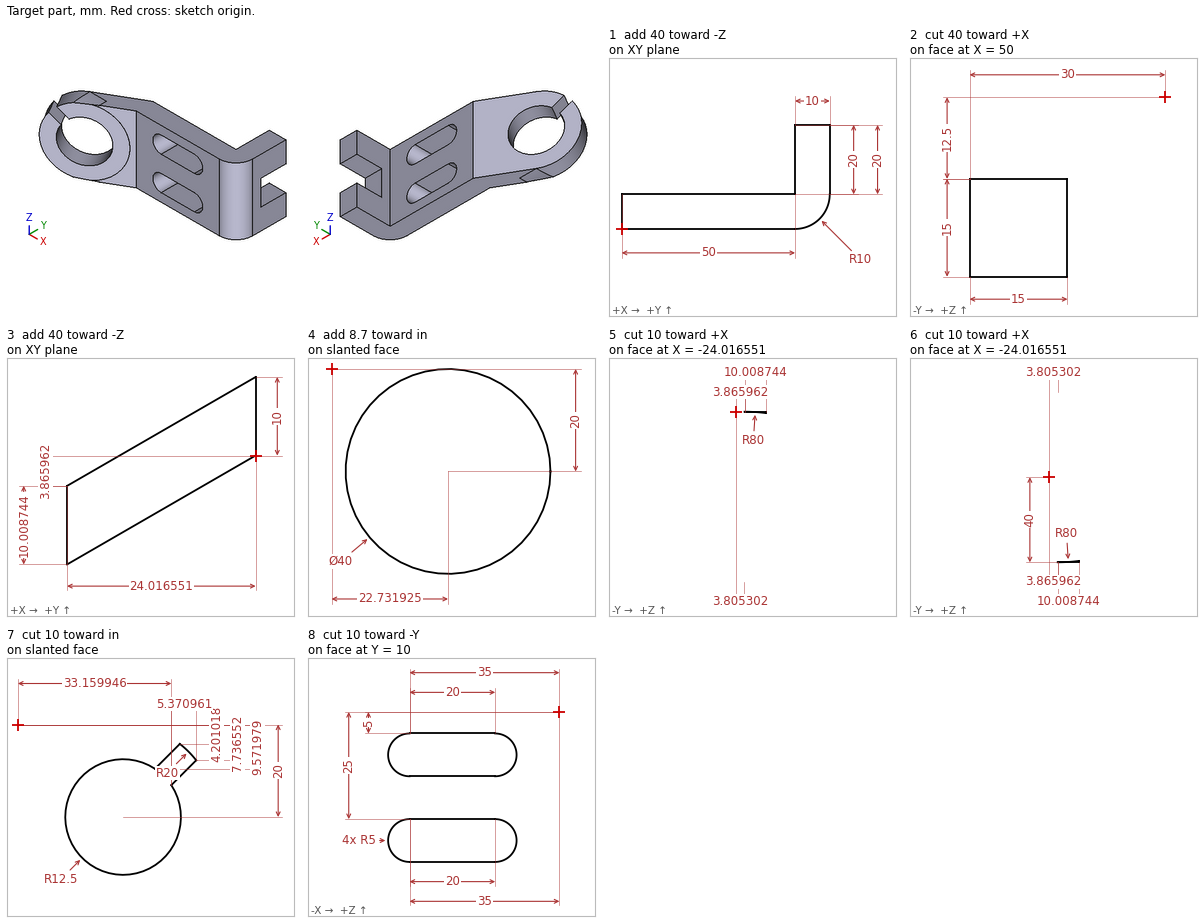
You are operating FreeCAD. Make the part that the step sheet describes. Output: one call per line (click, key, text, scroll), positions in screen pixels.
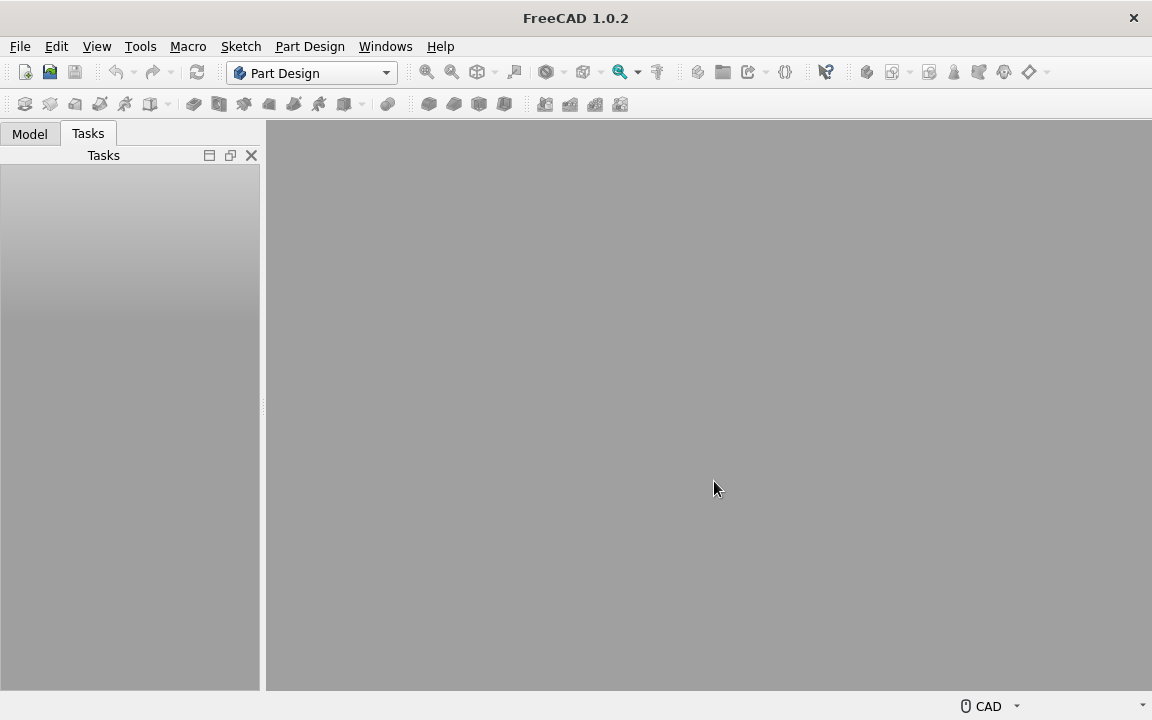
click(25, 72)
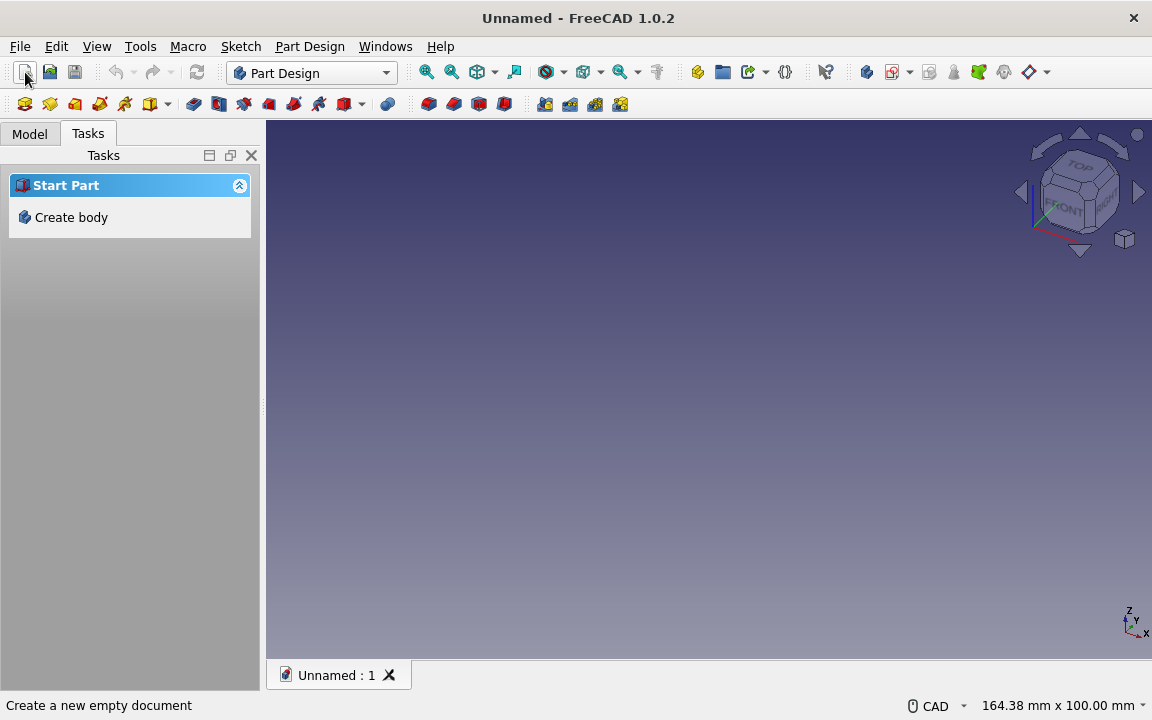
click(892, 72)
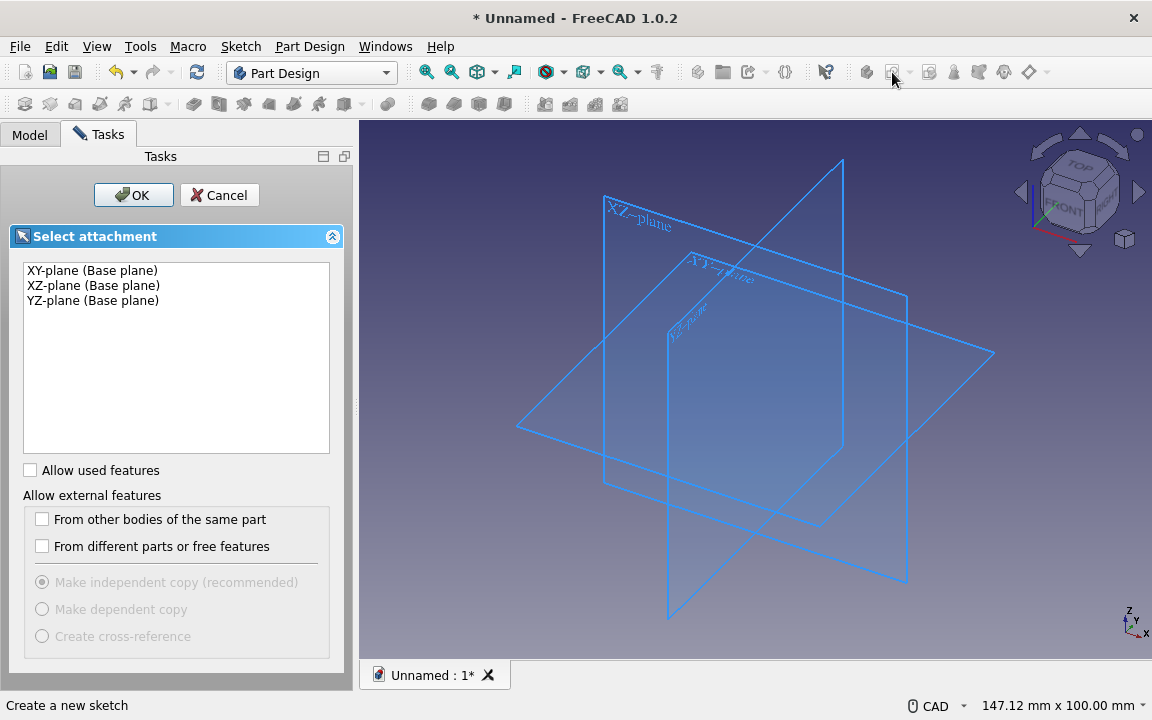
click(84, 270)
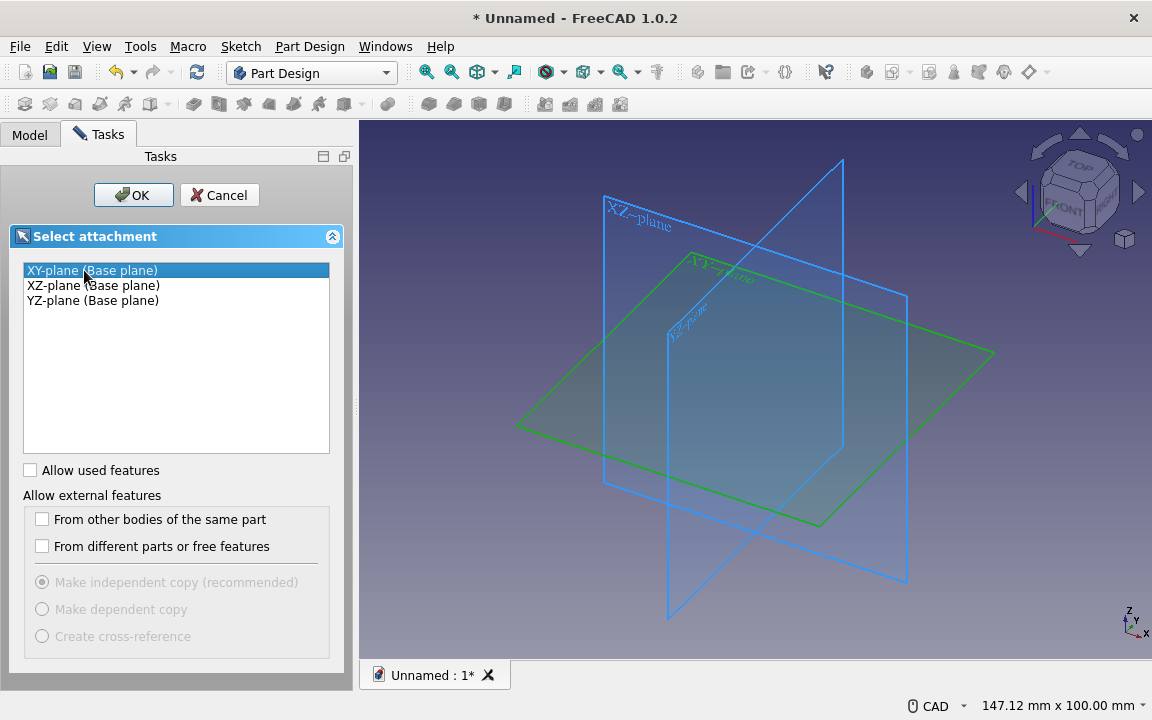
click(134, 195)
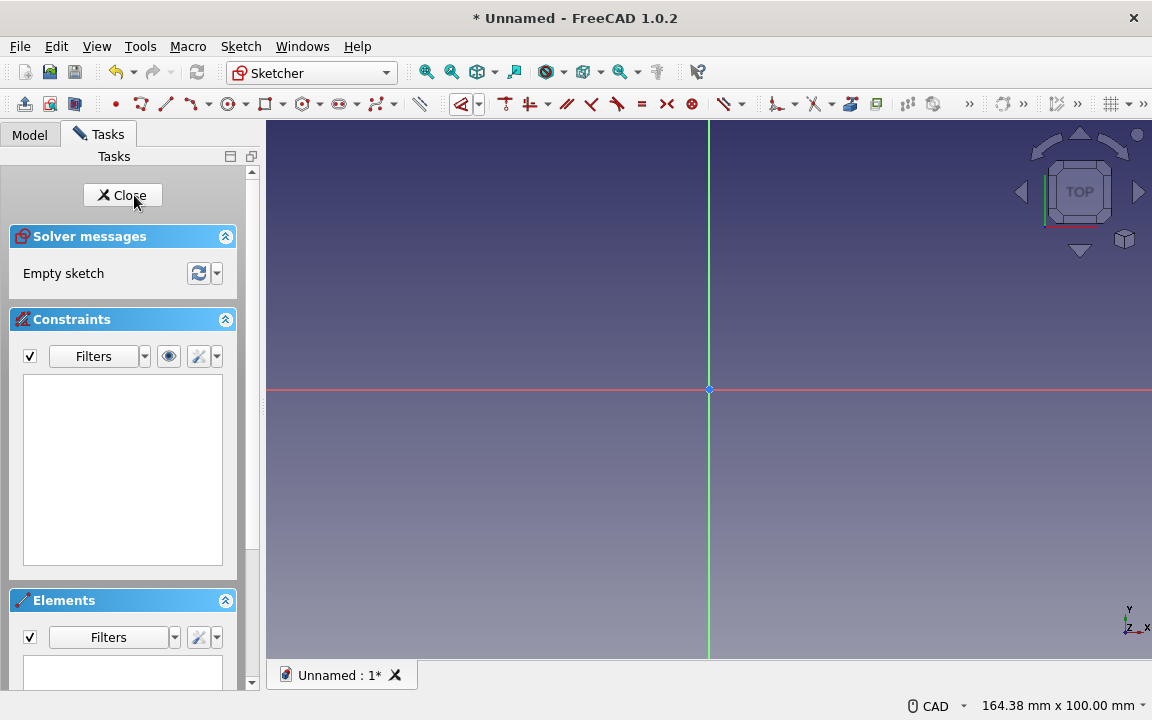
scroll(294, 631, down, 1)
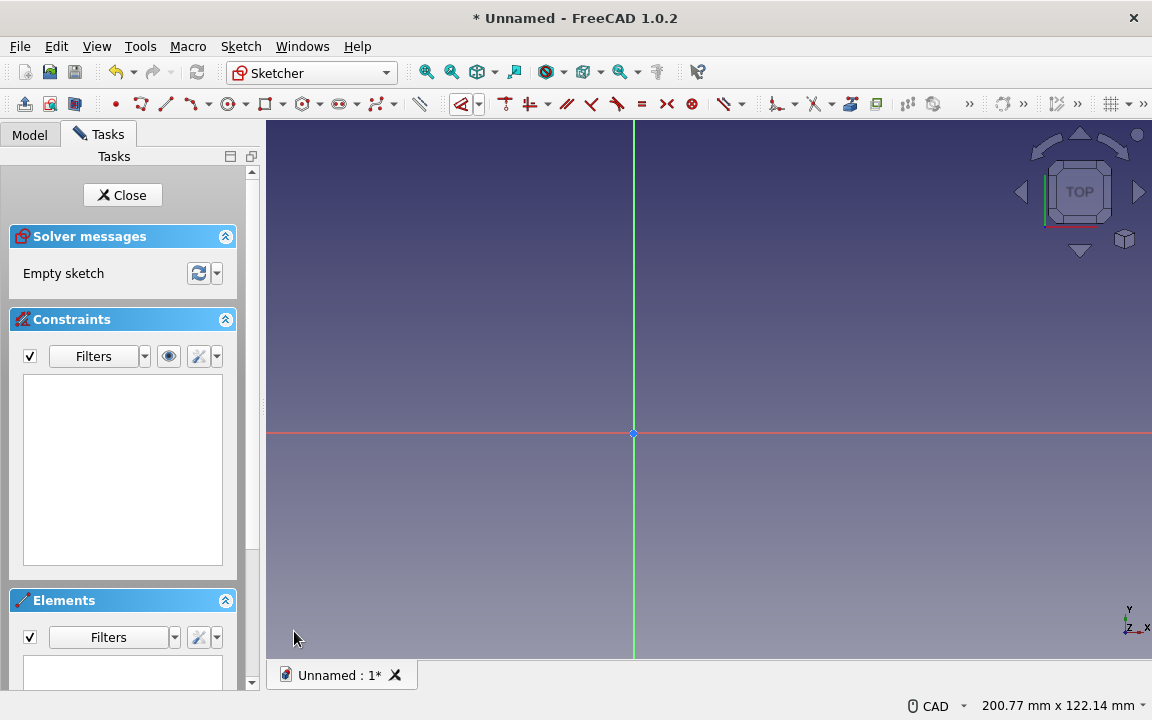
scroll(919, 340, up, 3)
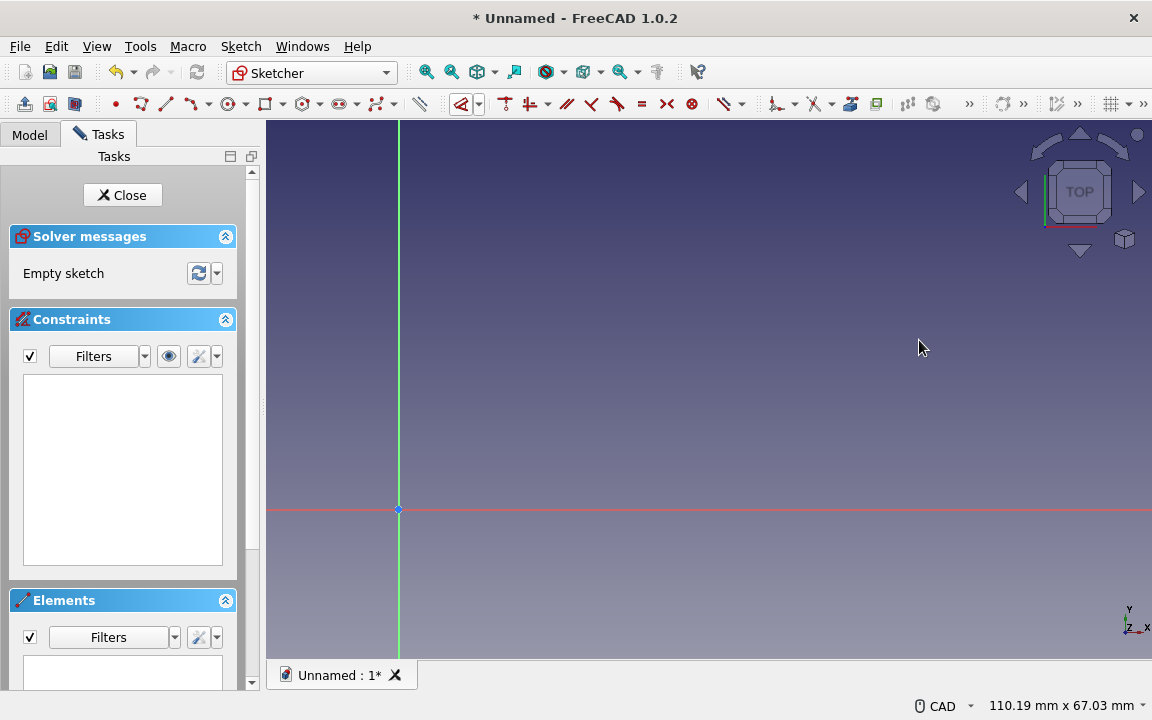
click(141, 104)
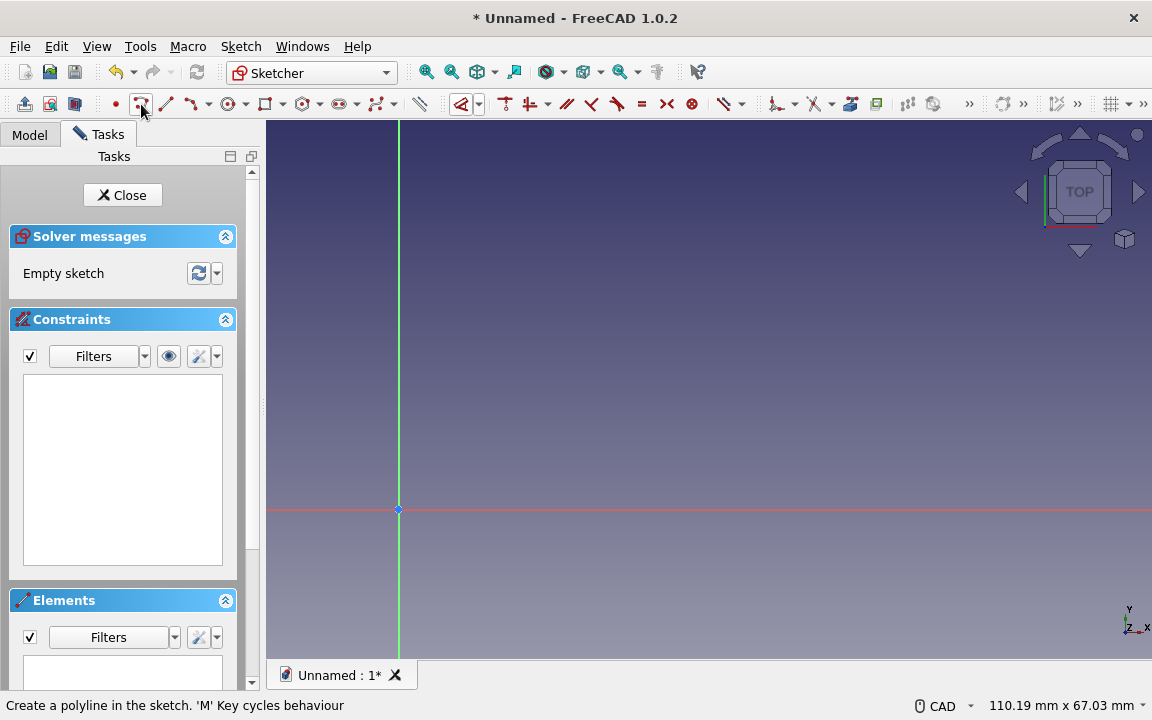
click(881, 430)
click(881, 269)
click(801, 269)
click(801, 430)
click(399, 430)
click(399, 510)
click(801, 501)
right_click(801, 501)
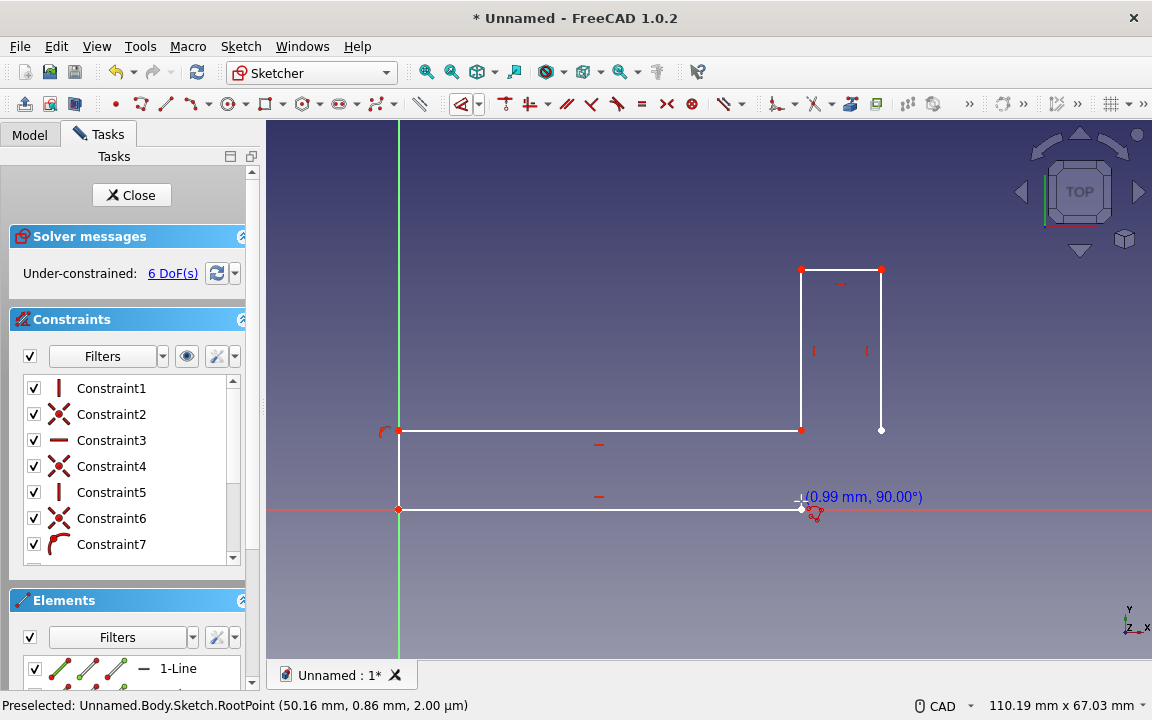
click(190, 104)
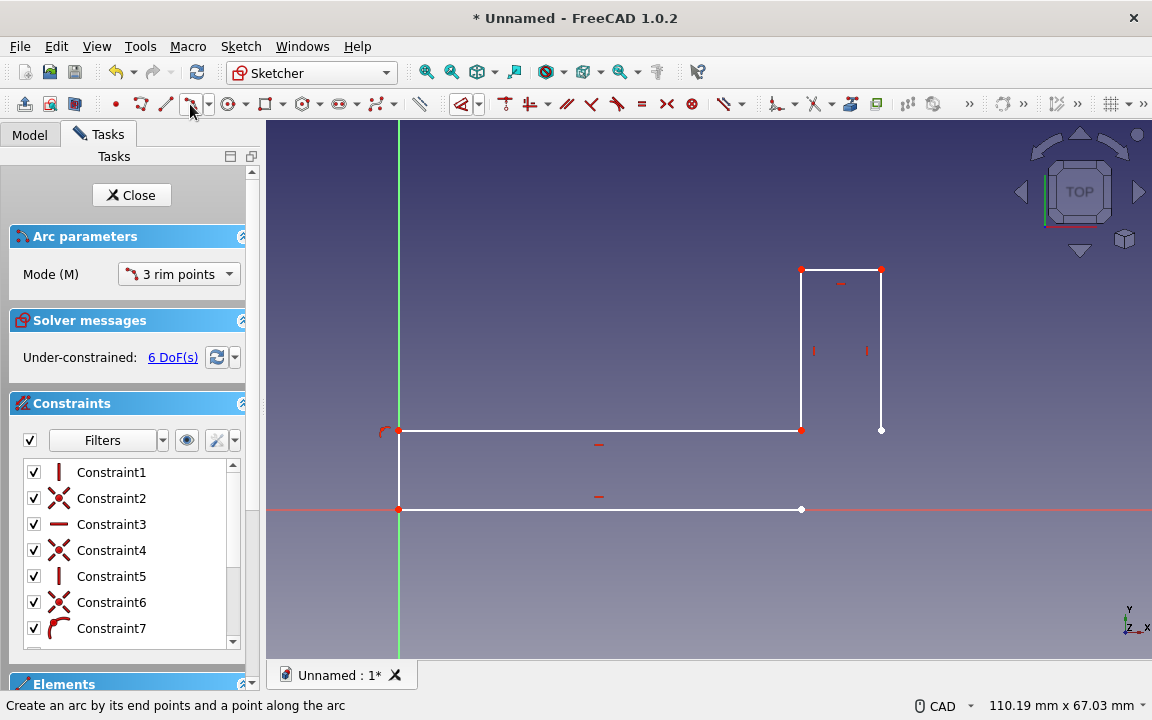
click(801, 510)
click(881, 431)
click(858, 486)
key(Escape)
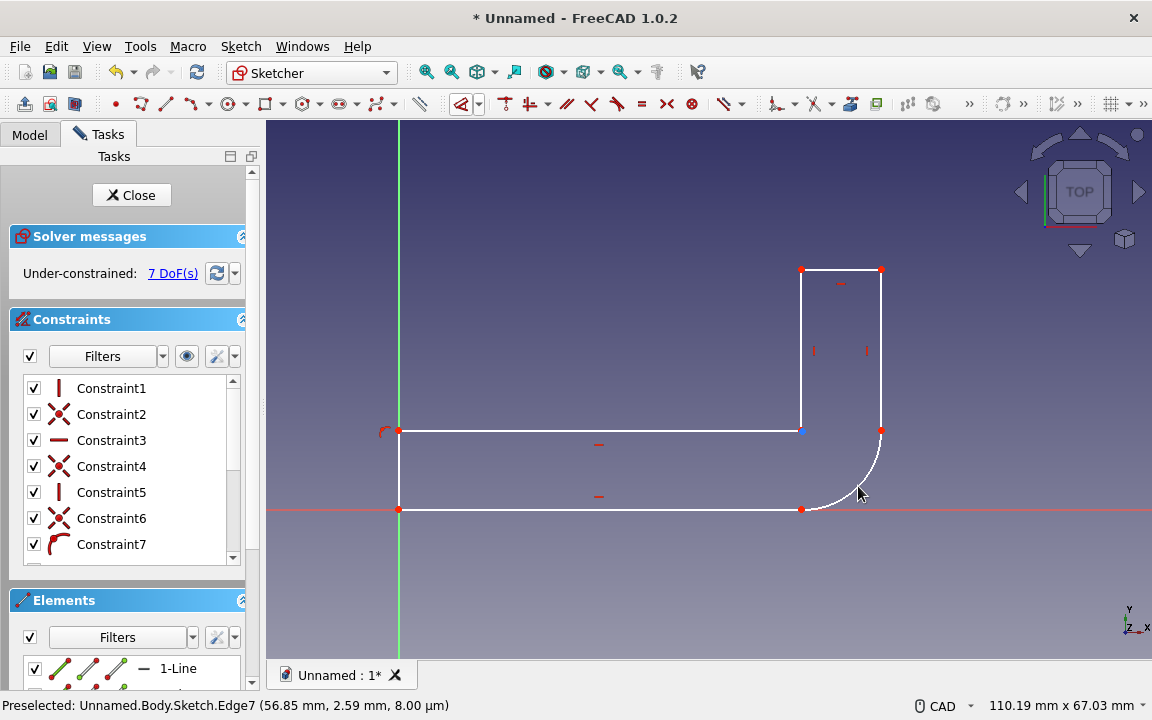
click(881, 383)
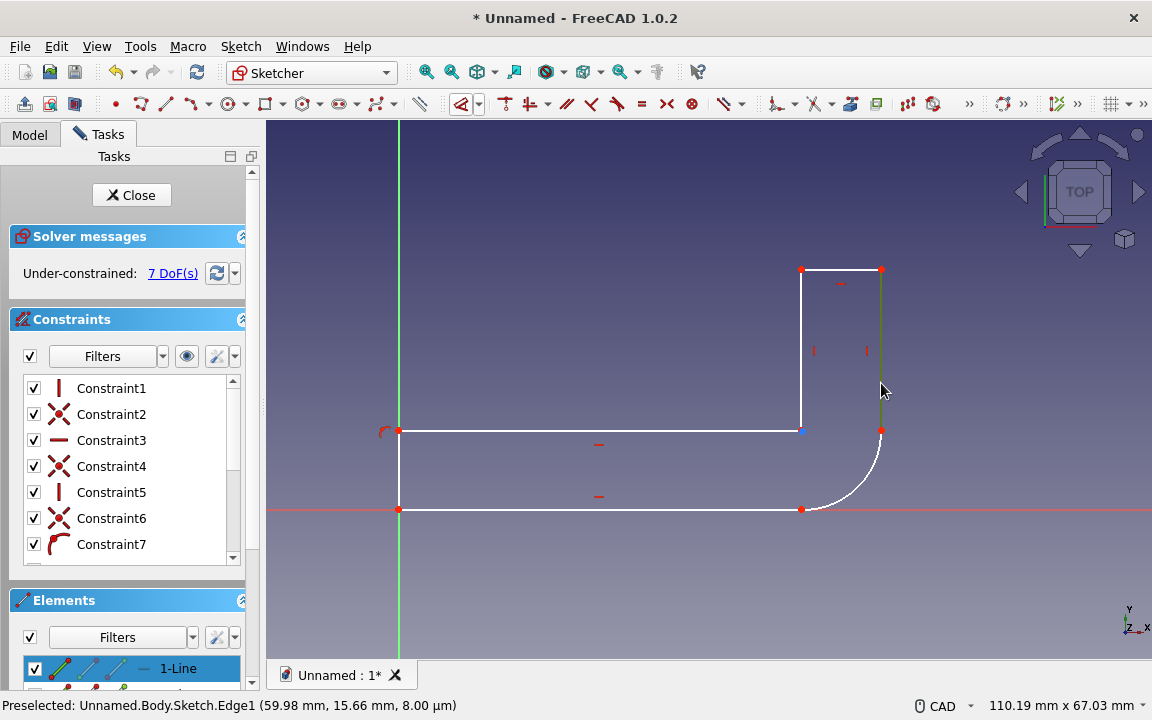
click(872, 467)